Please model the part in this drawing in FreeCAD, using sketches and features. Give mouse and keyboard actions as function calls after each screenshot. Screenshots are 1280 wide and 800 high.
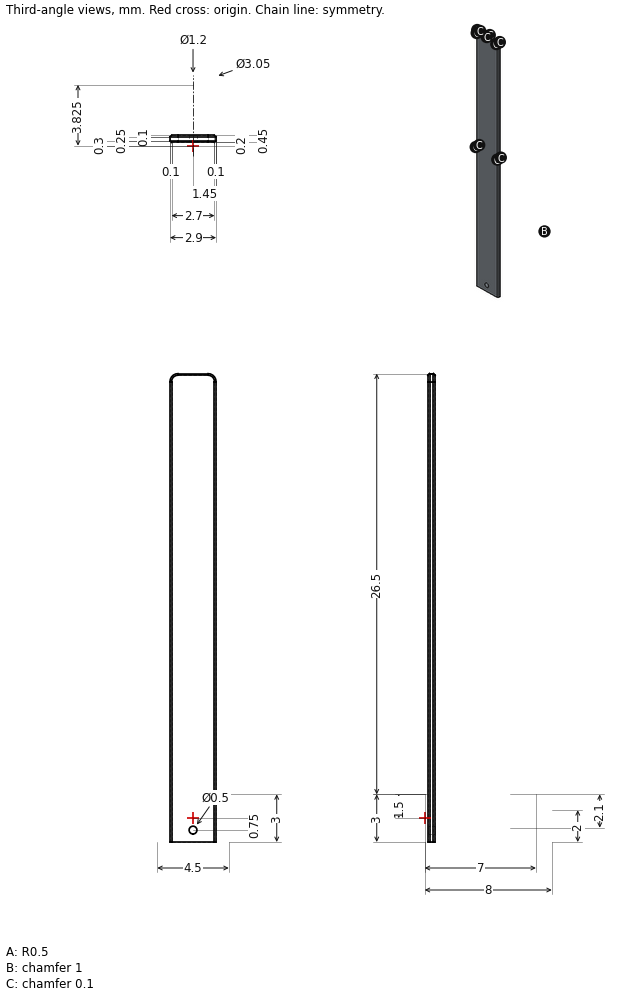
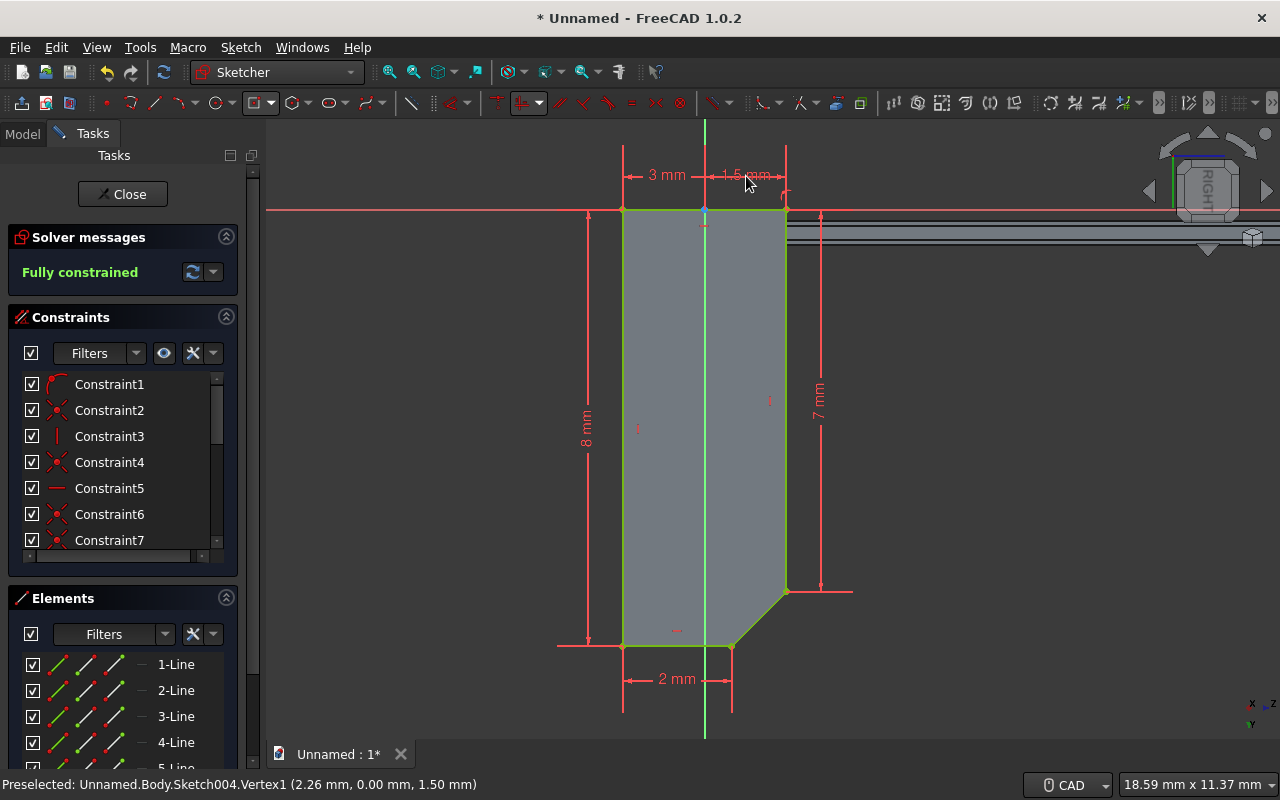
click(123, 194)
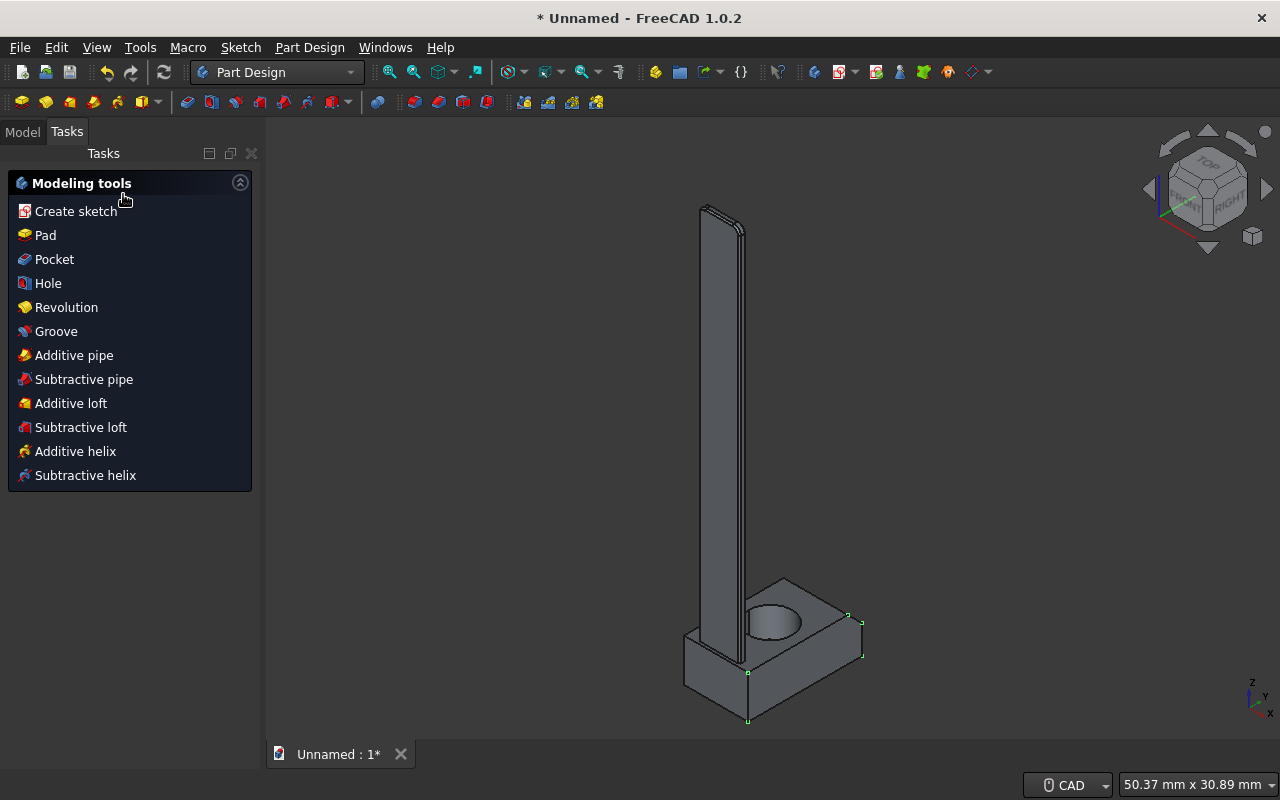
click(188, 102)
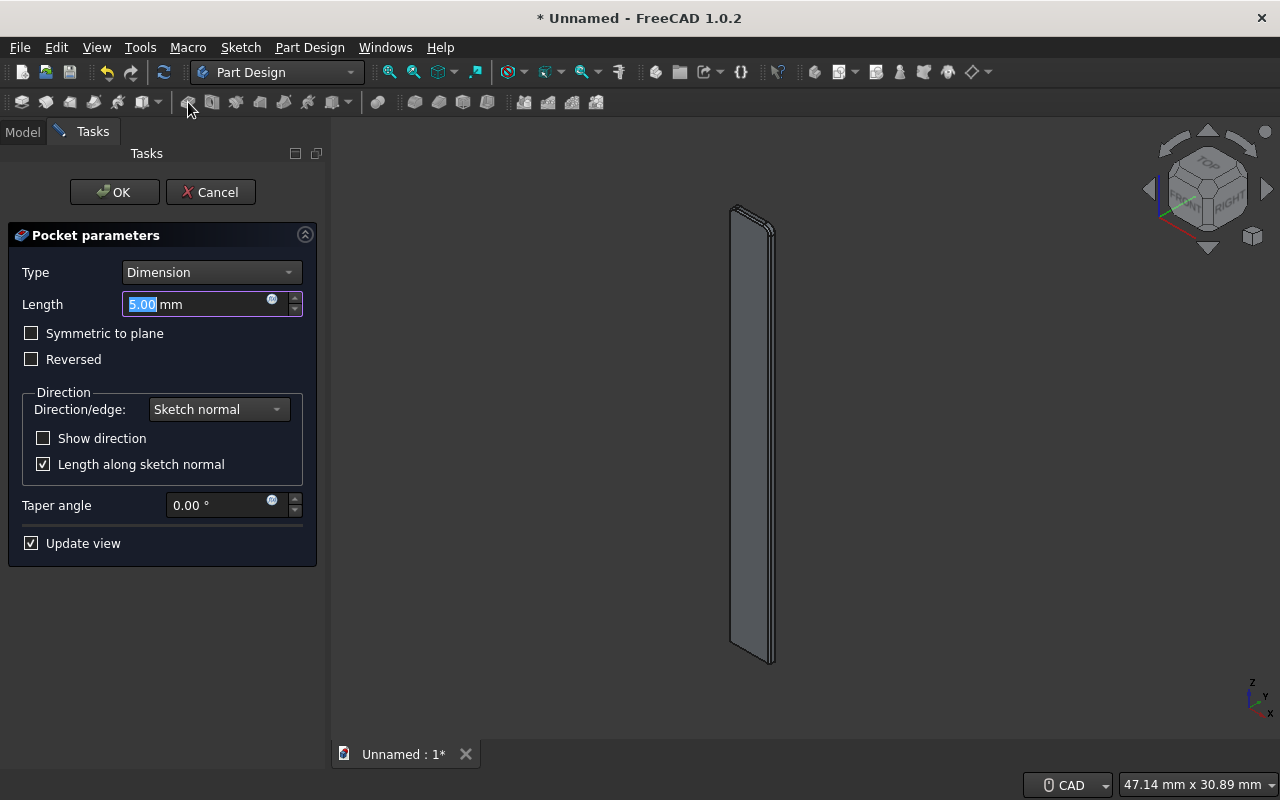
click(212, 272)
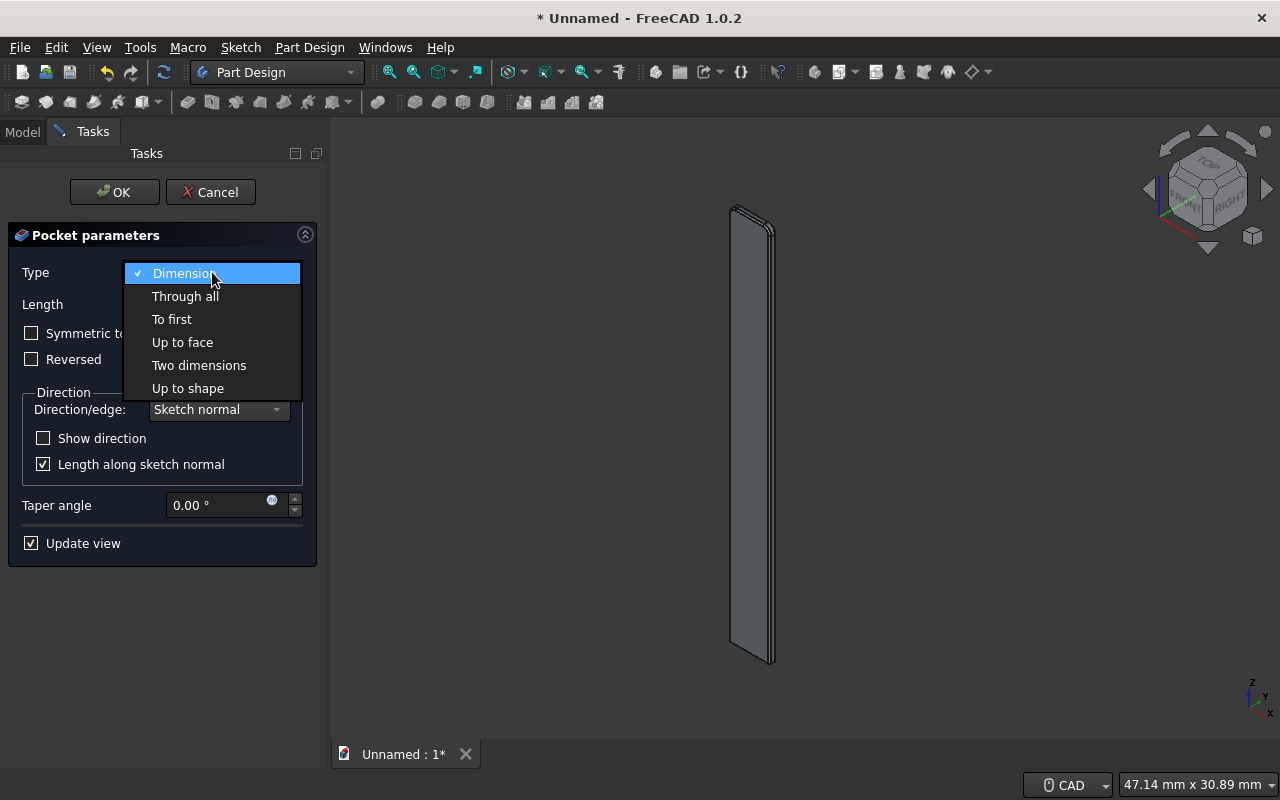
click(212, 296)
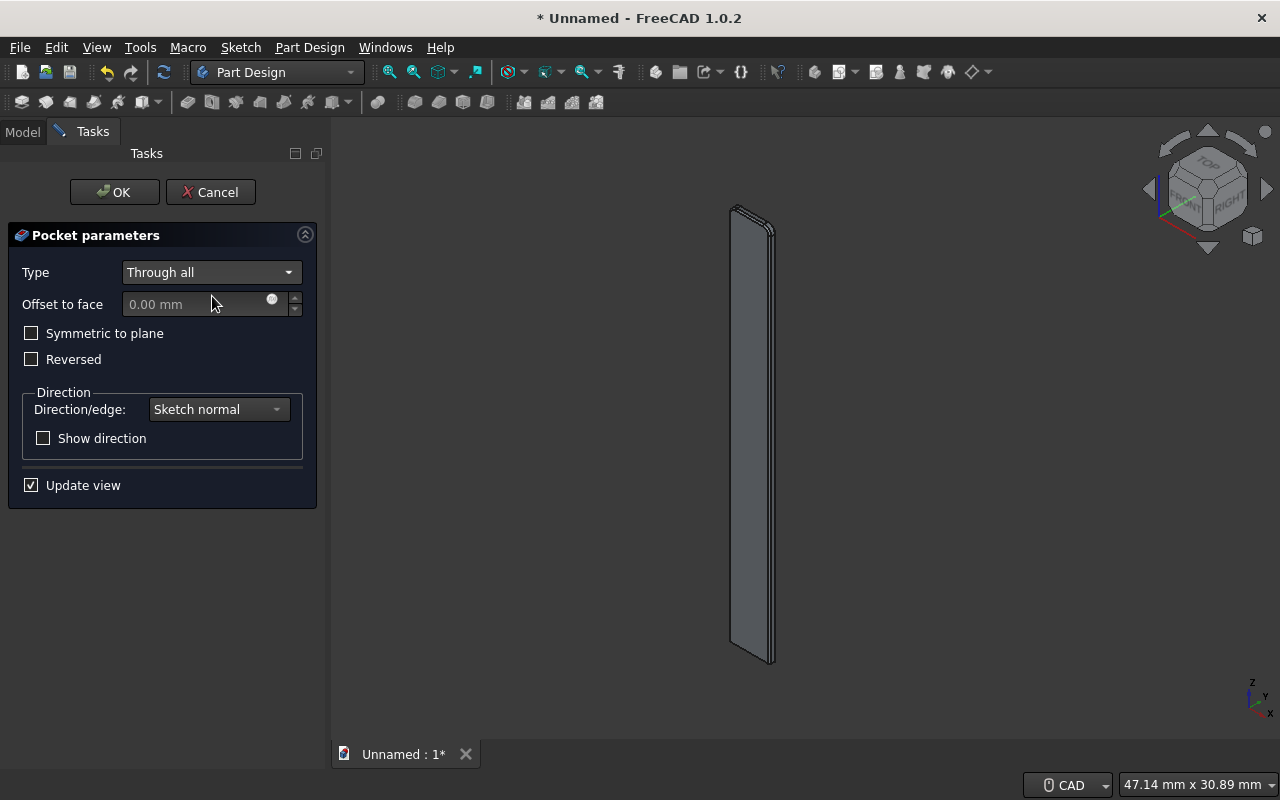
click(115, 192)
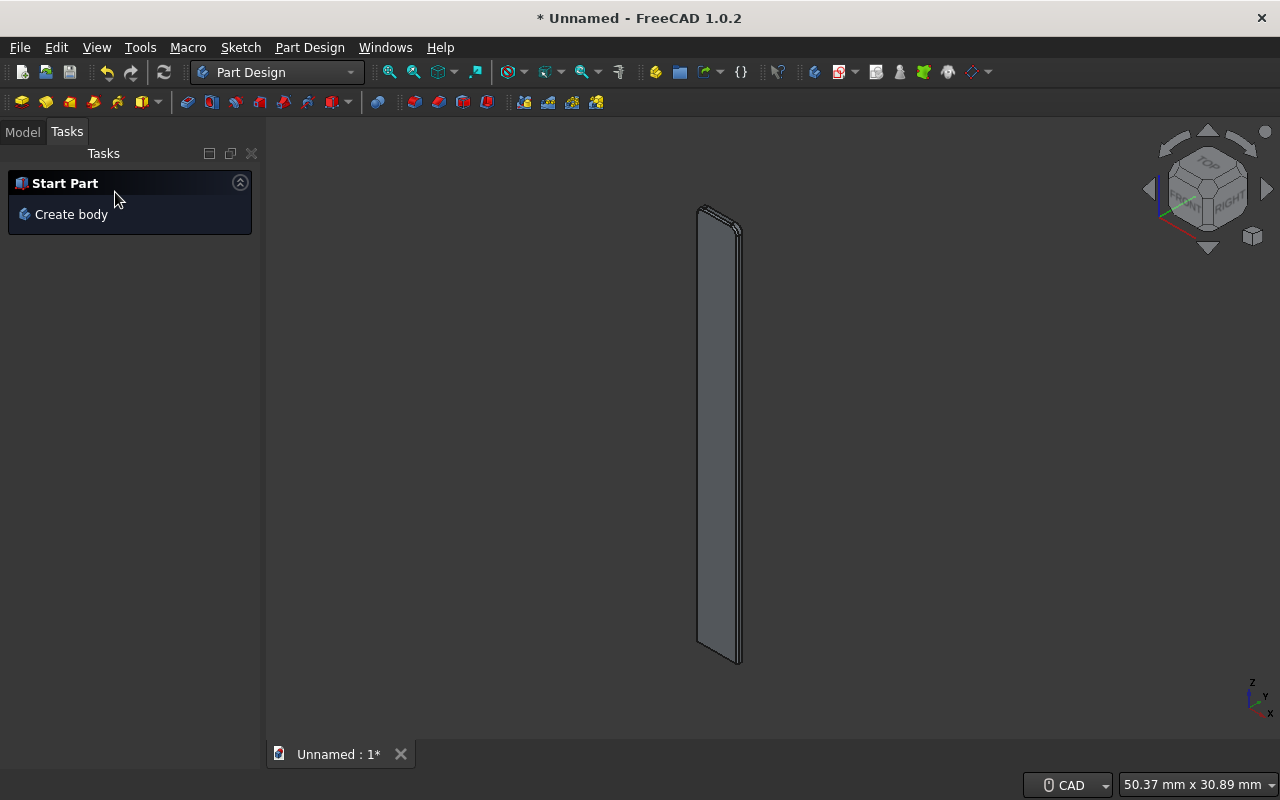
key(5)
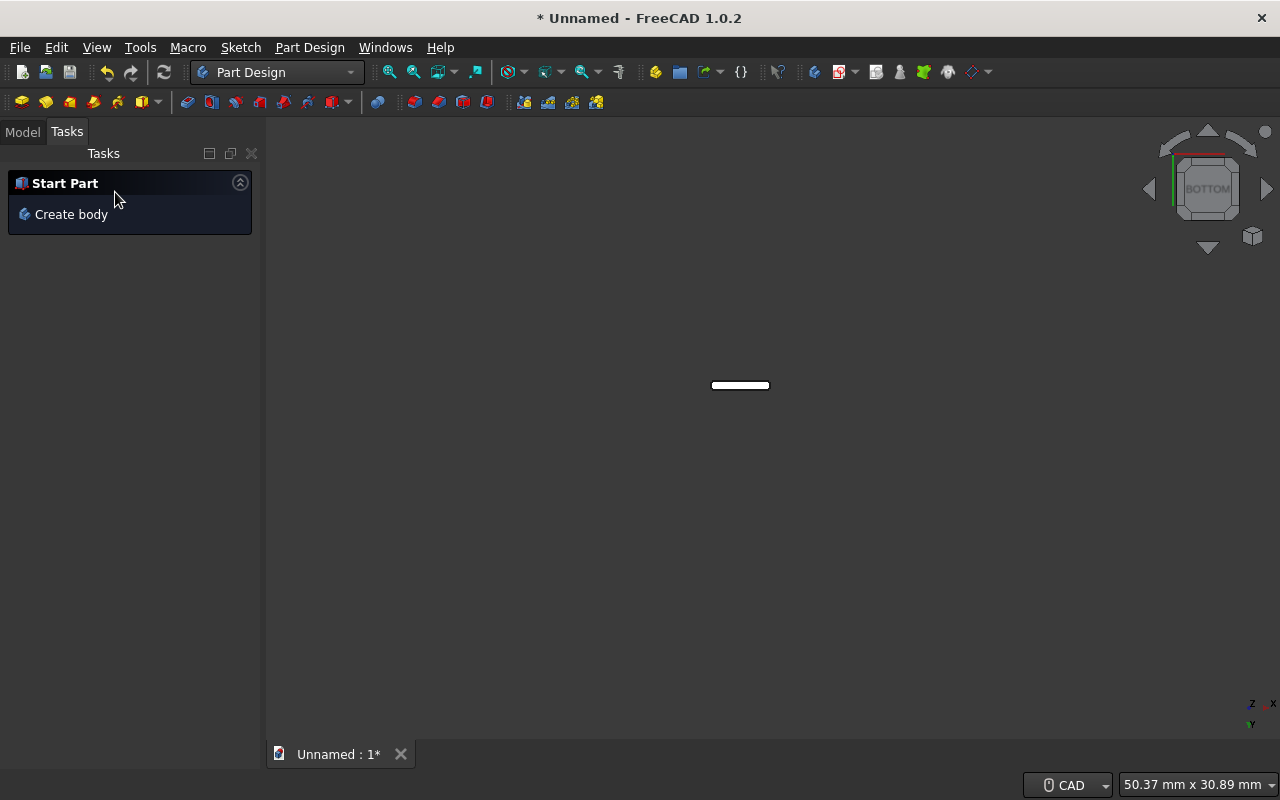
key(v)
key(f)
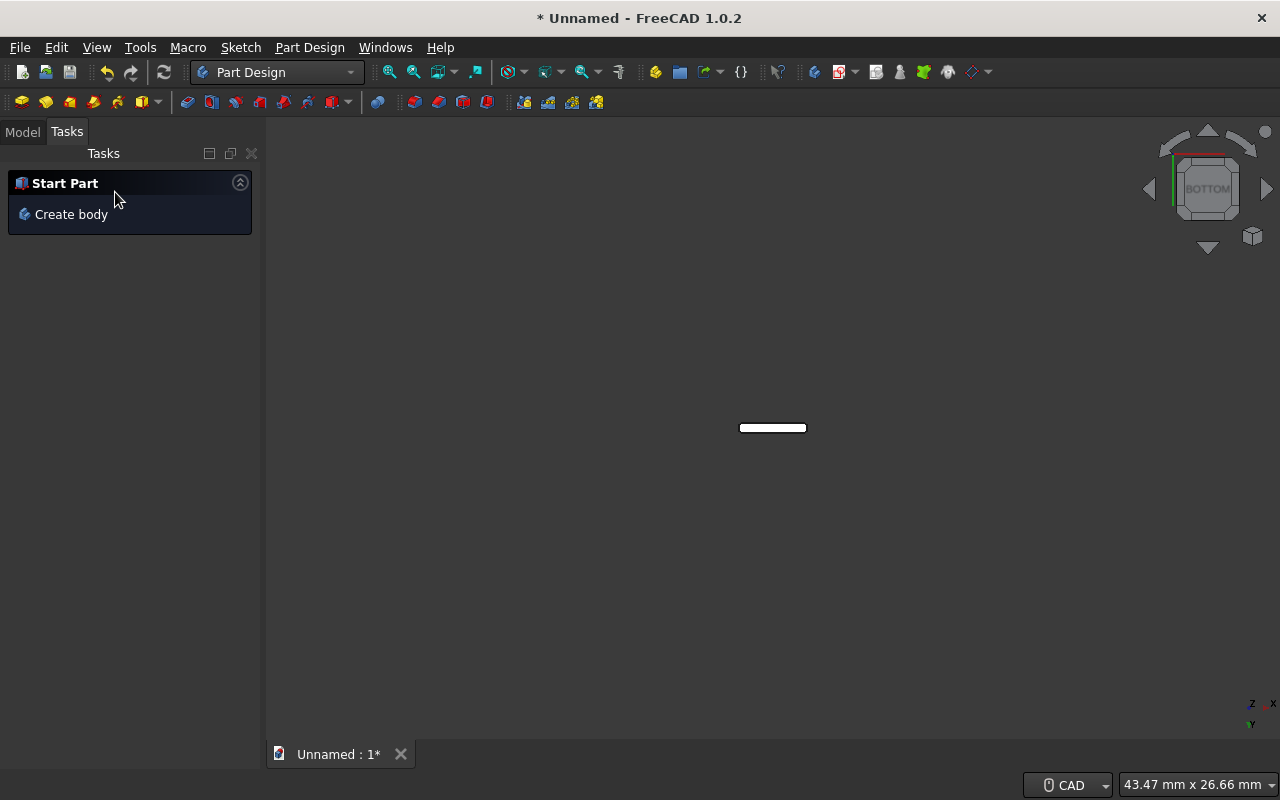
scroll(792, 427, up, 5)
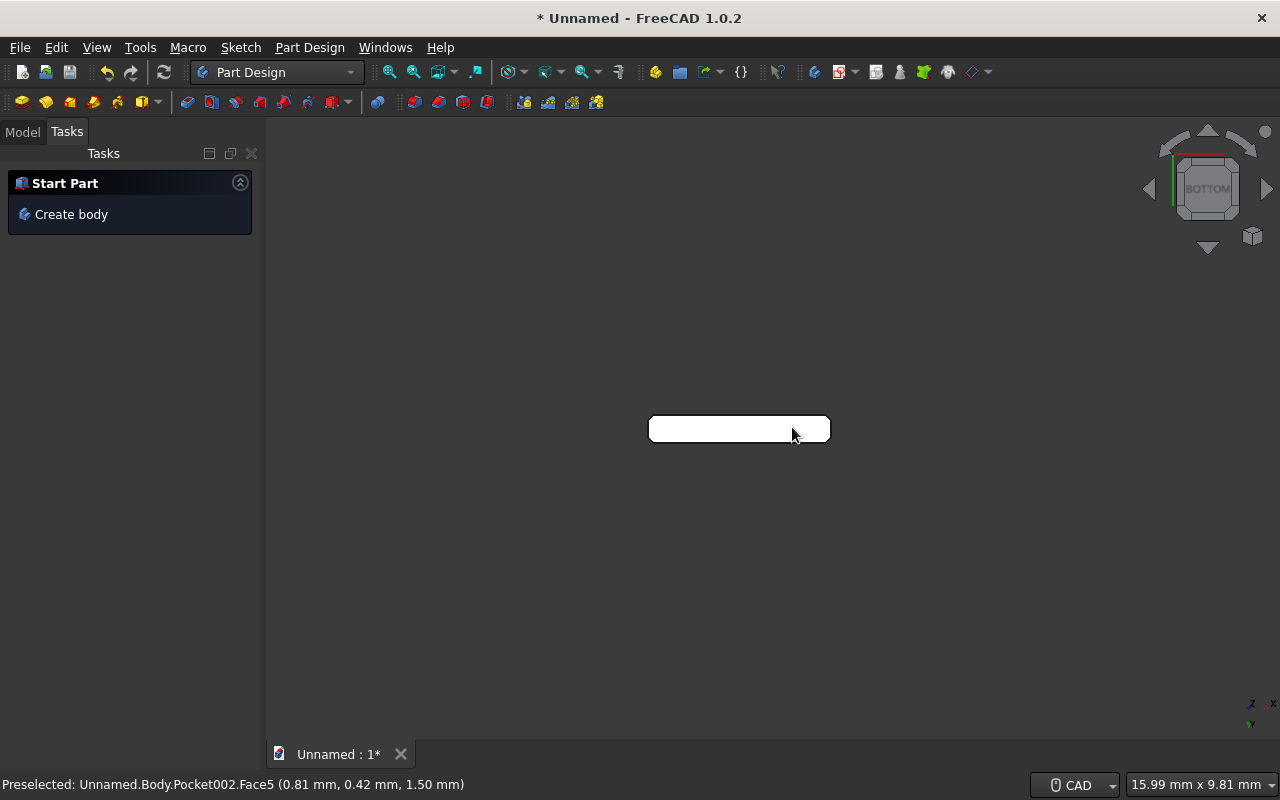
click(792, 428)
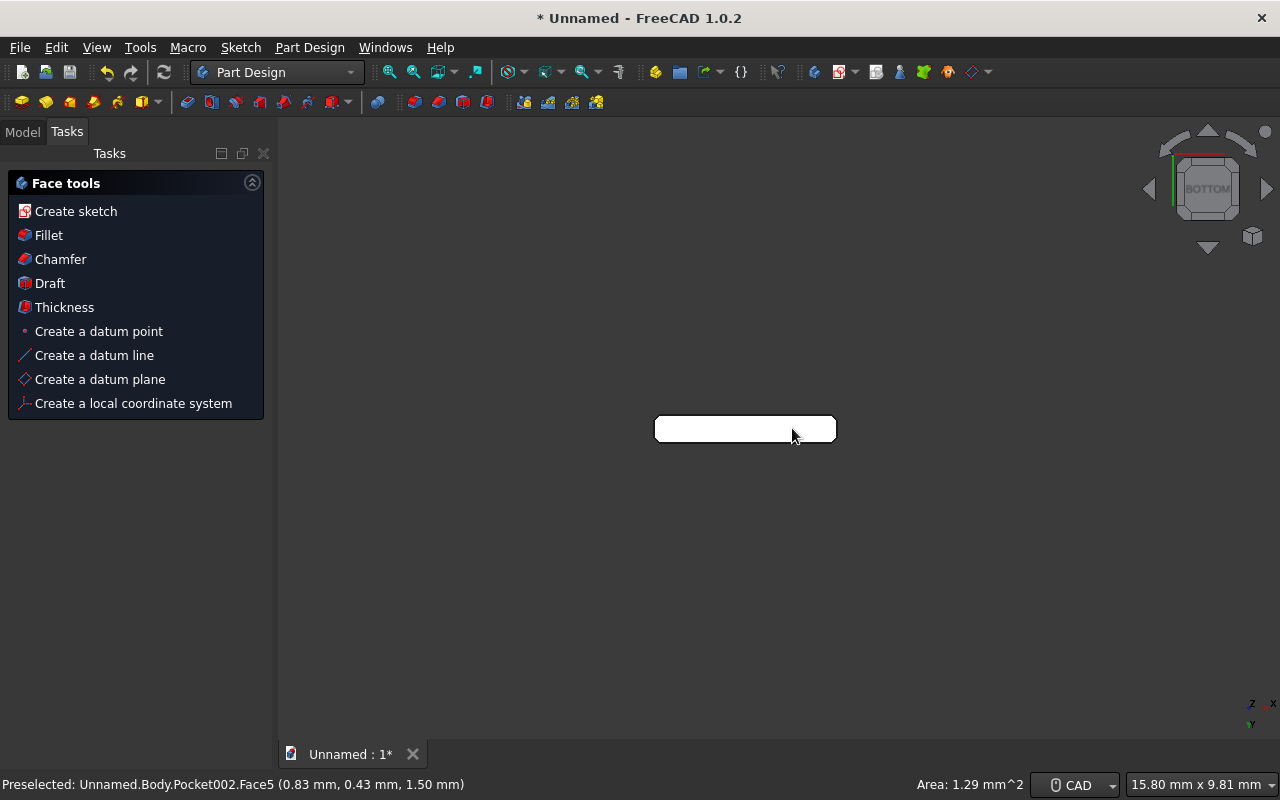
click(840, 72)